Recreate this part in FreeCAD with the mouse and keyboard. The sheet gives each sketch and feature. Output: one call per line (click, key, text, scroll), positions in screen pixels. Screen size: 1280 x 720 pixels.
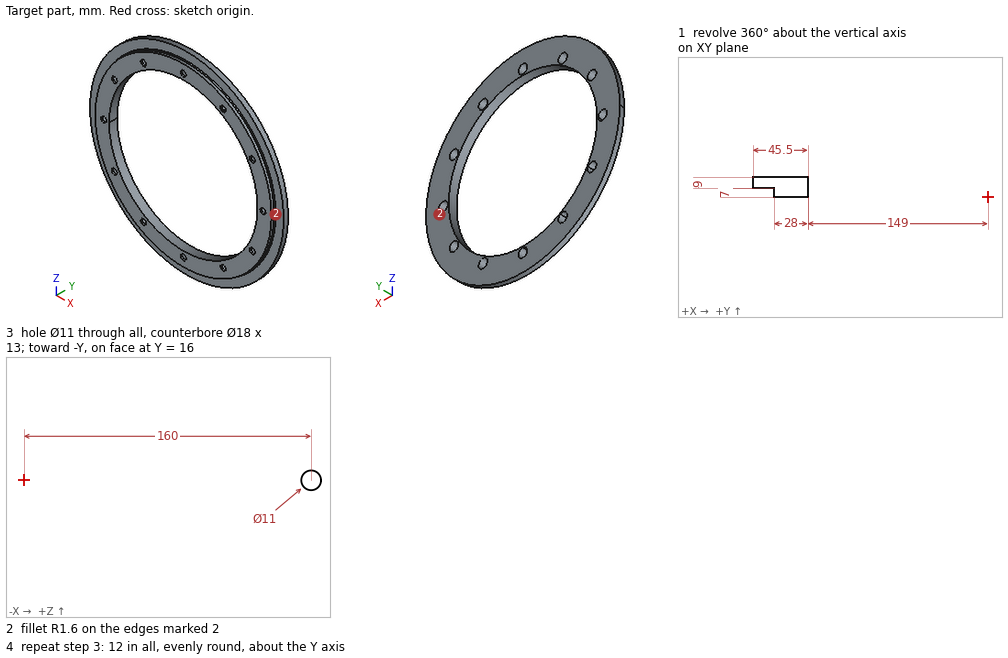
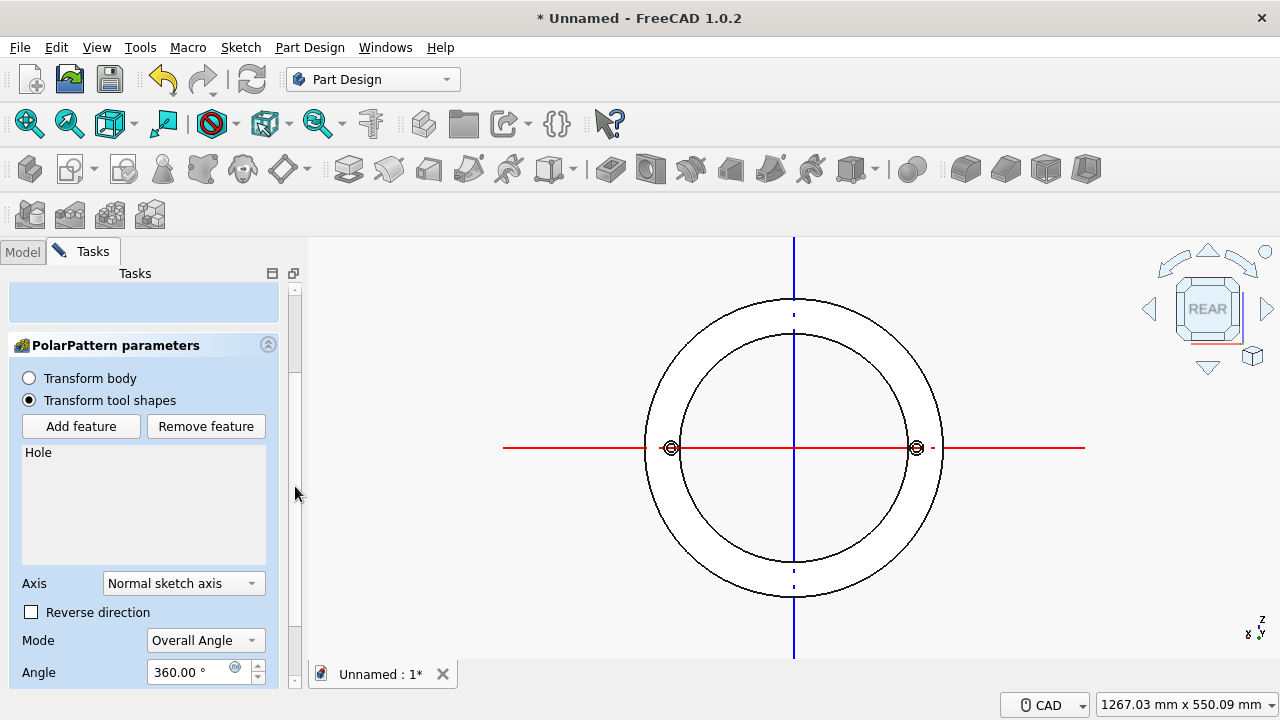
click(184, 584)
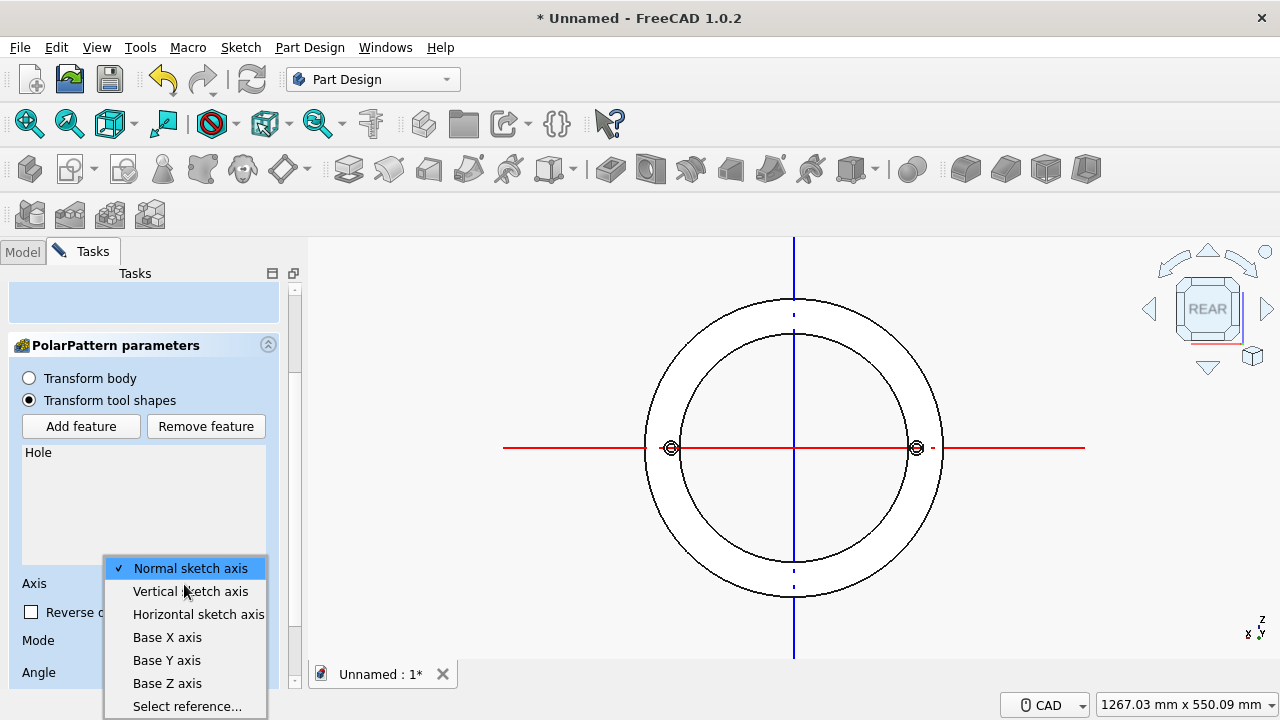
click(184, 660)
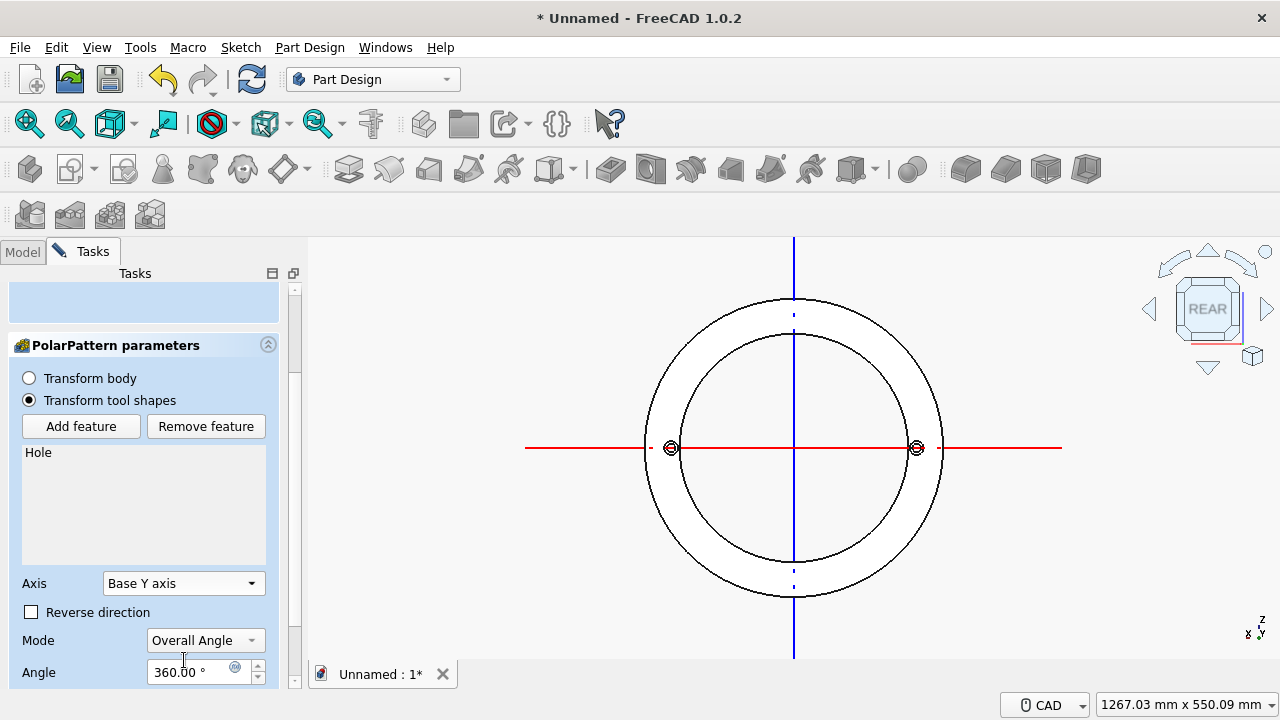
scroll(295, 486, down, 2)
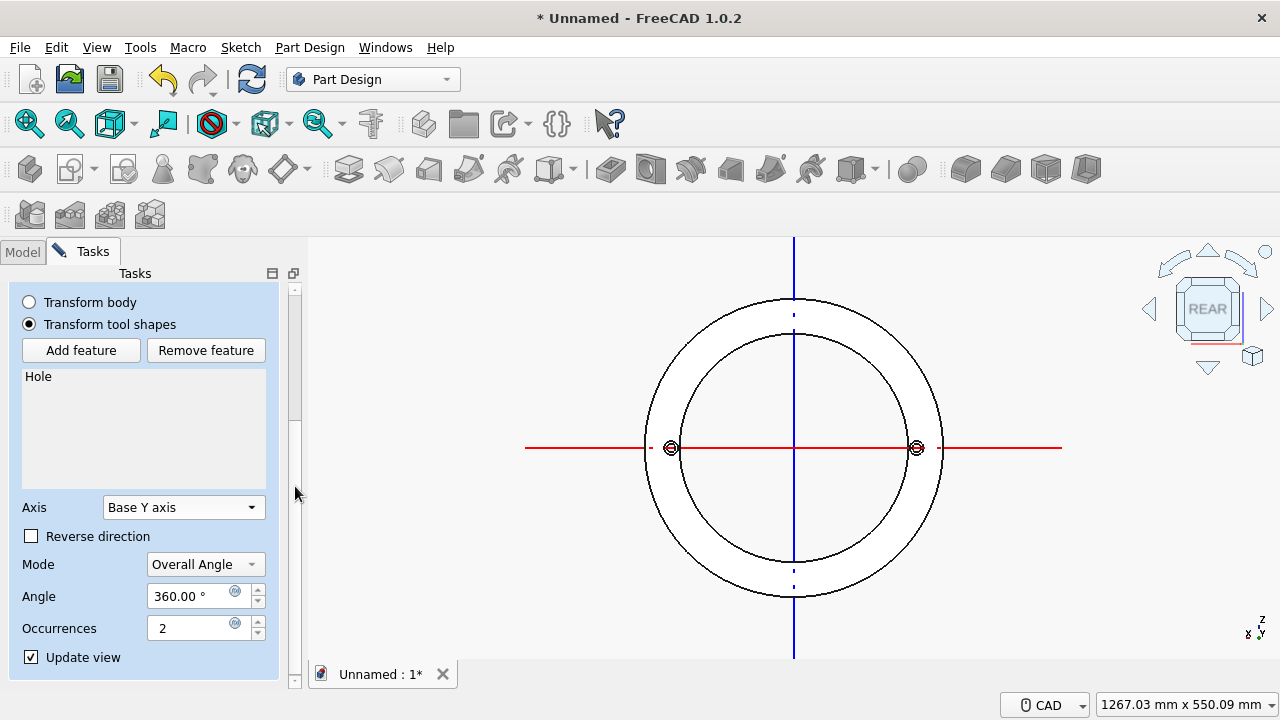
triple_click(198, 628)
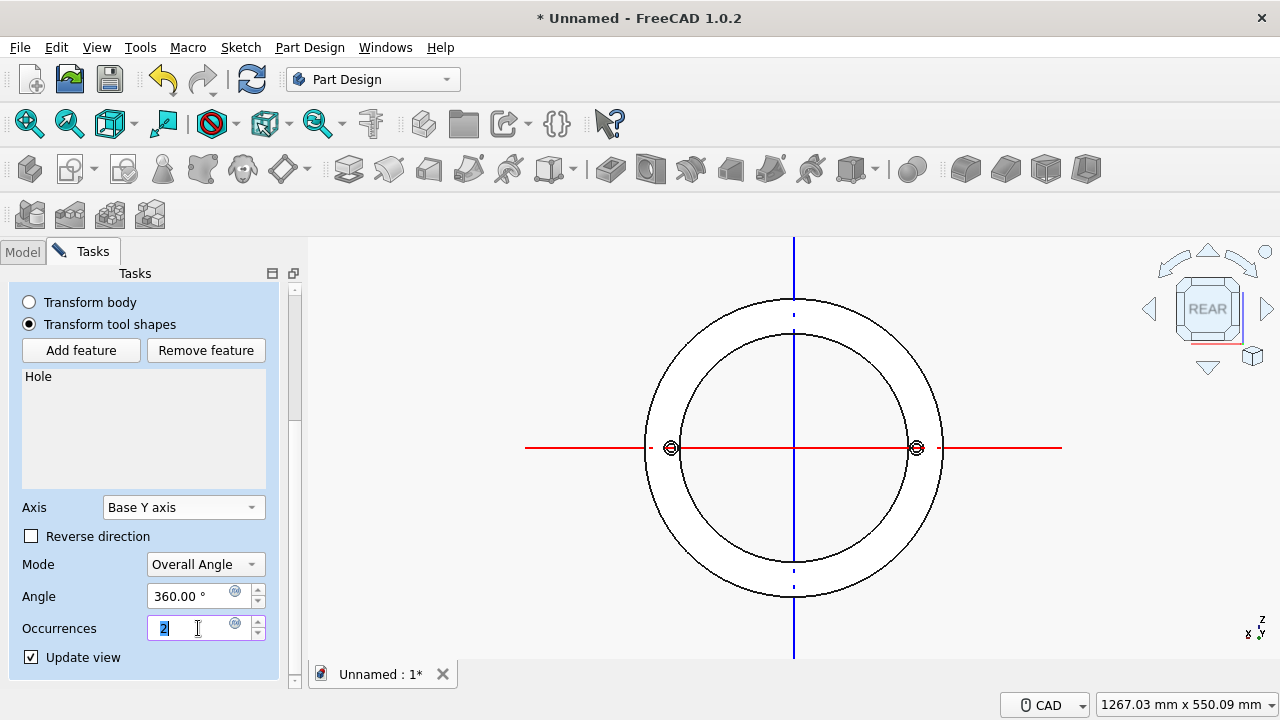
text(12)
key(Tab)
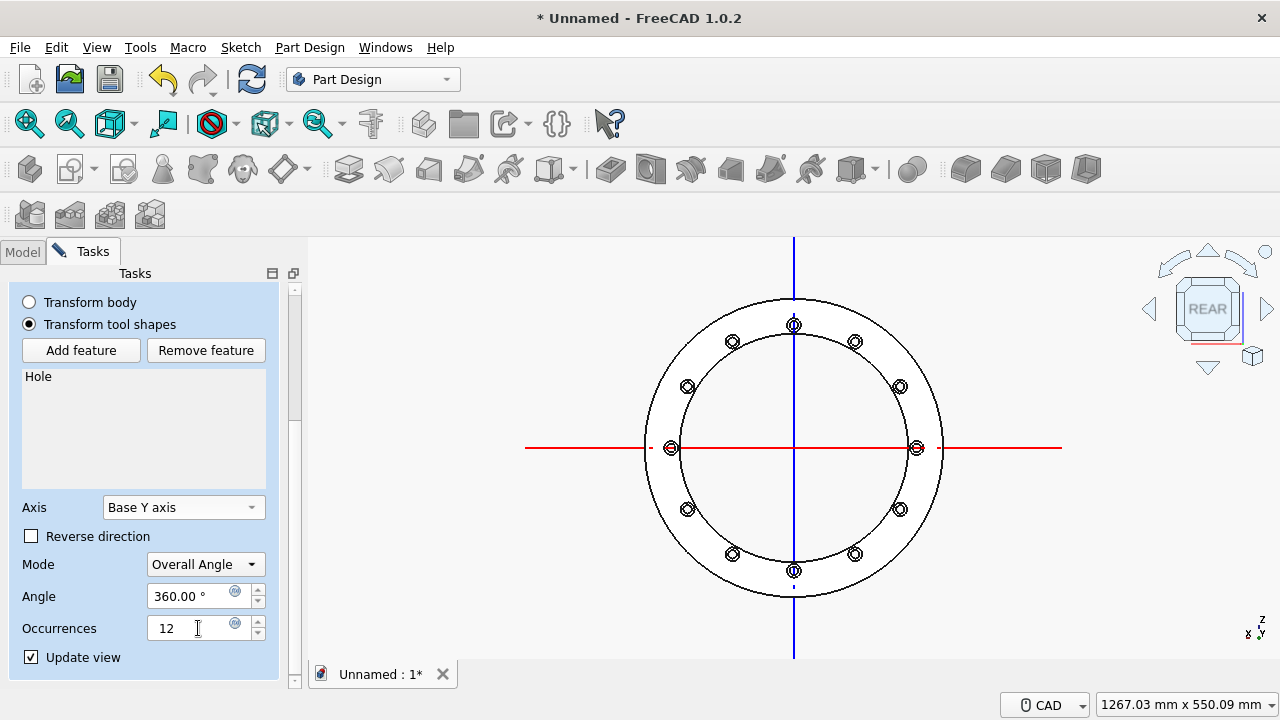
scroll(295, 486, up, 5)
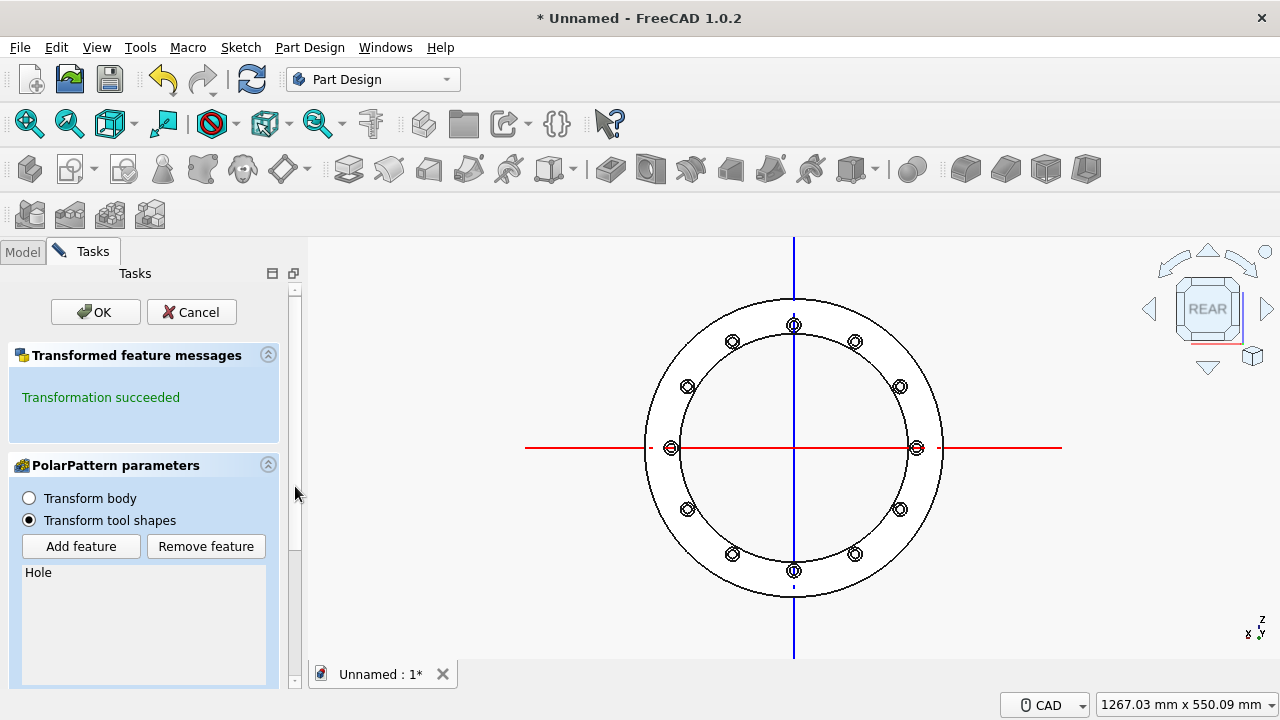
click(96, 312)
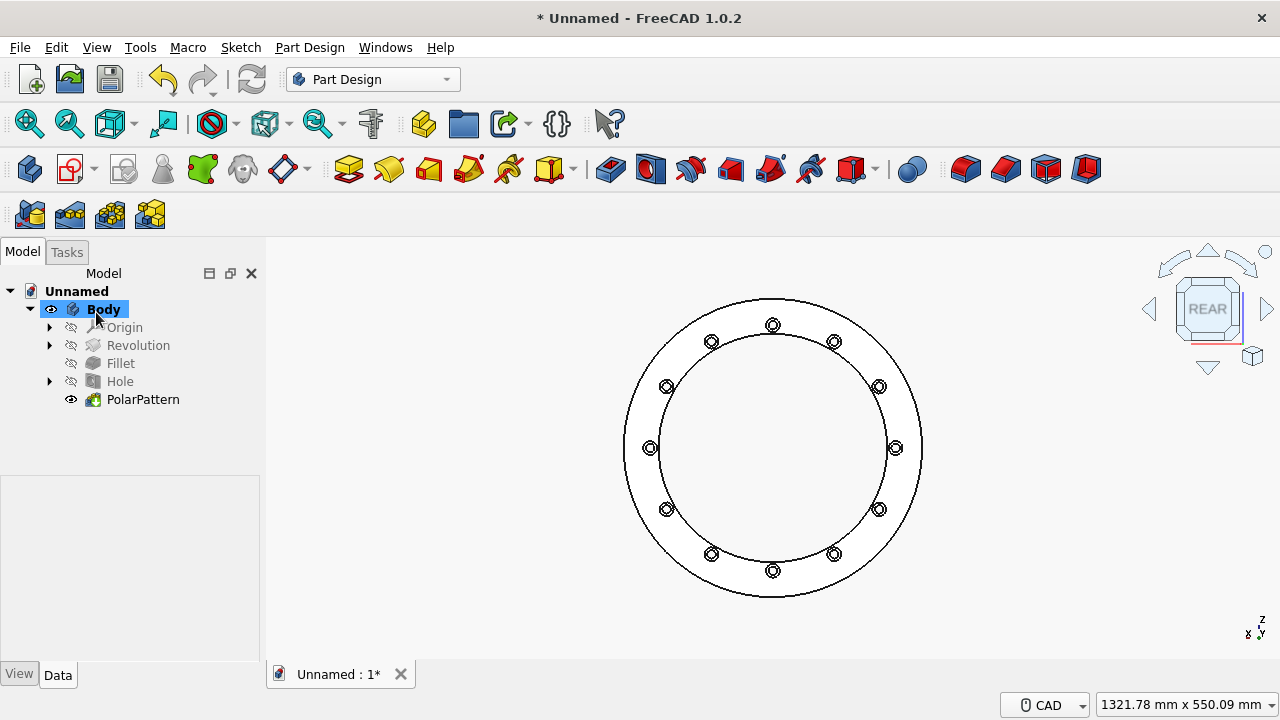
key(0)